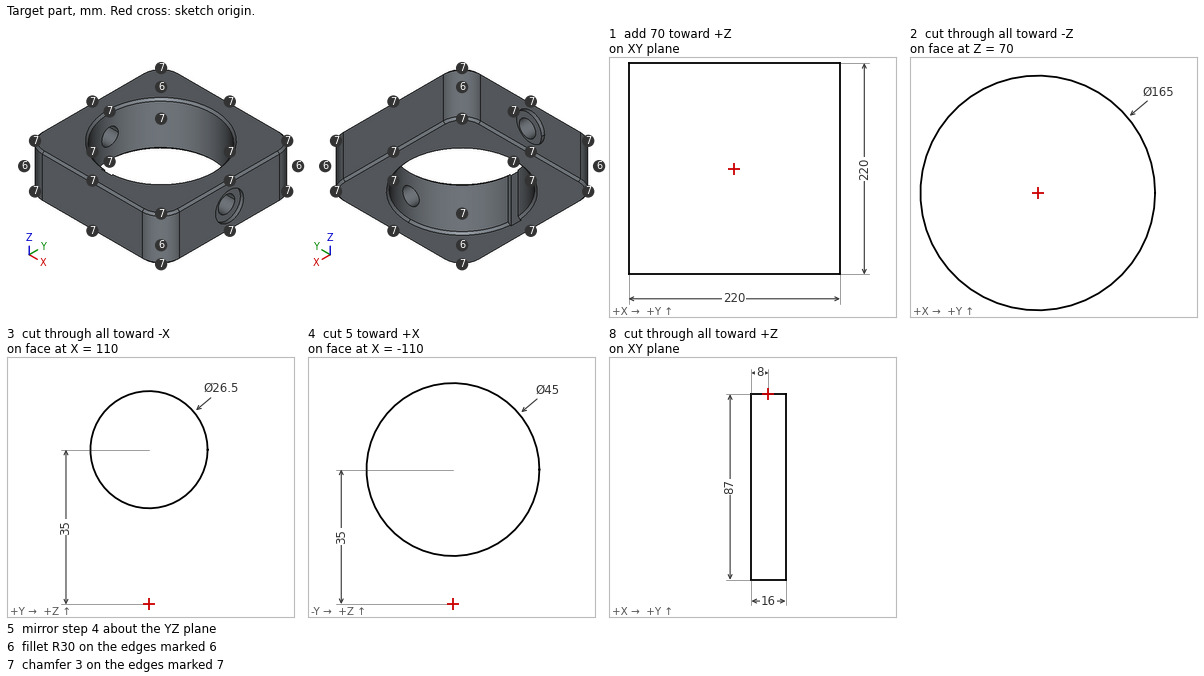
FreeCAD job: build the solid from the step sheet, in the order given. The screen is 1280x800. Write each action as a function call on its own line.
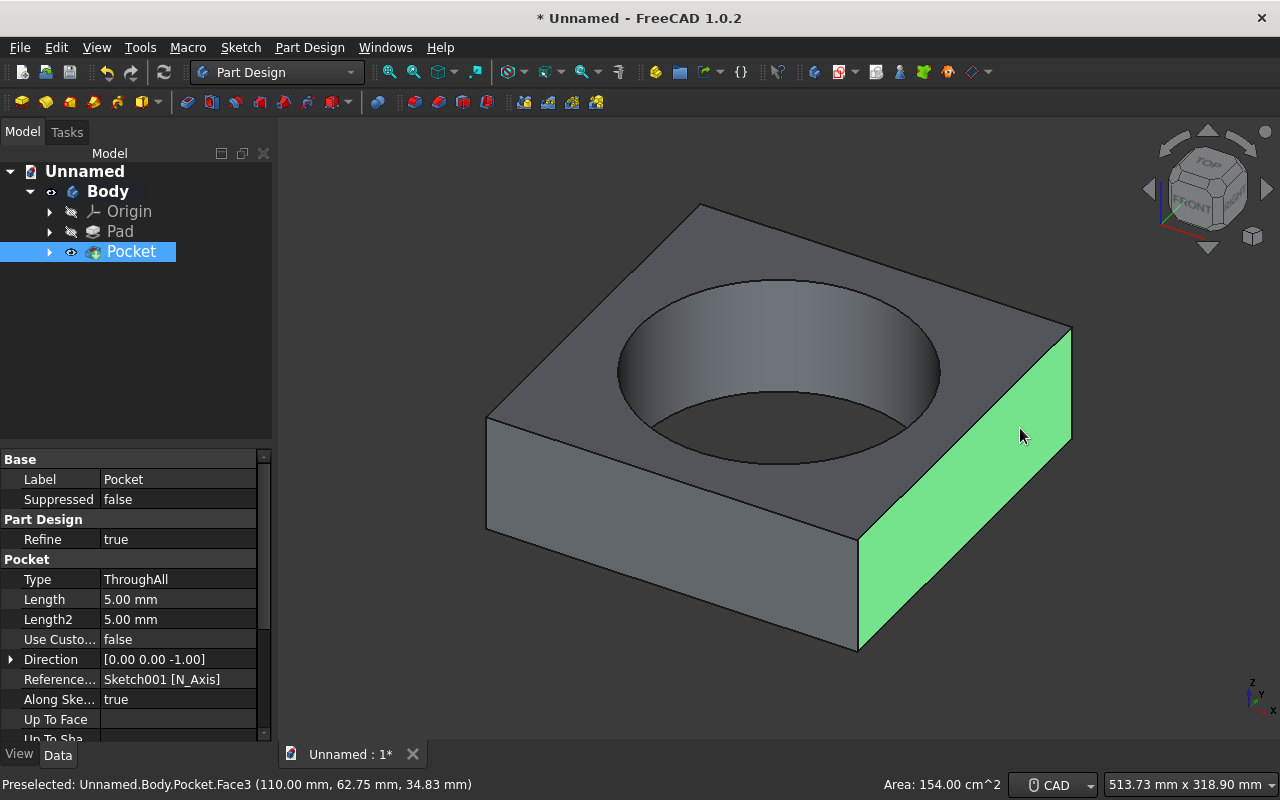
click(840, 72)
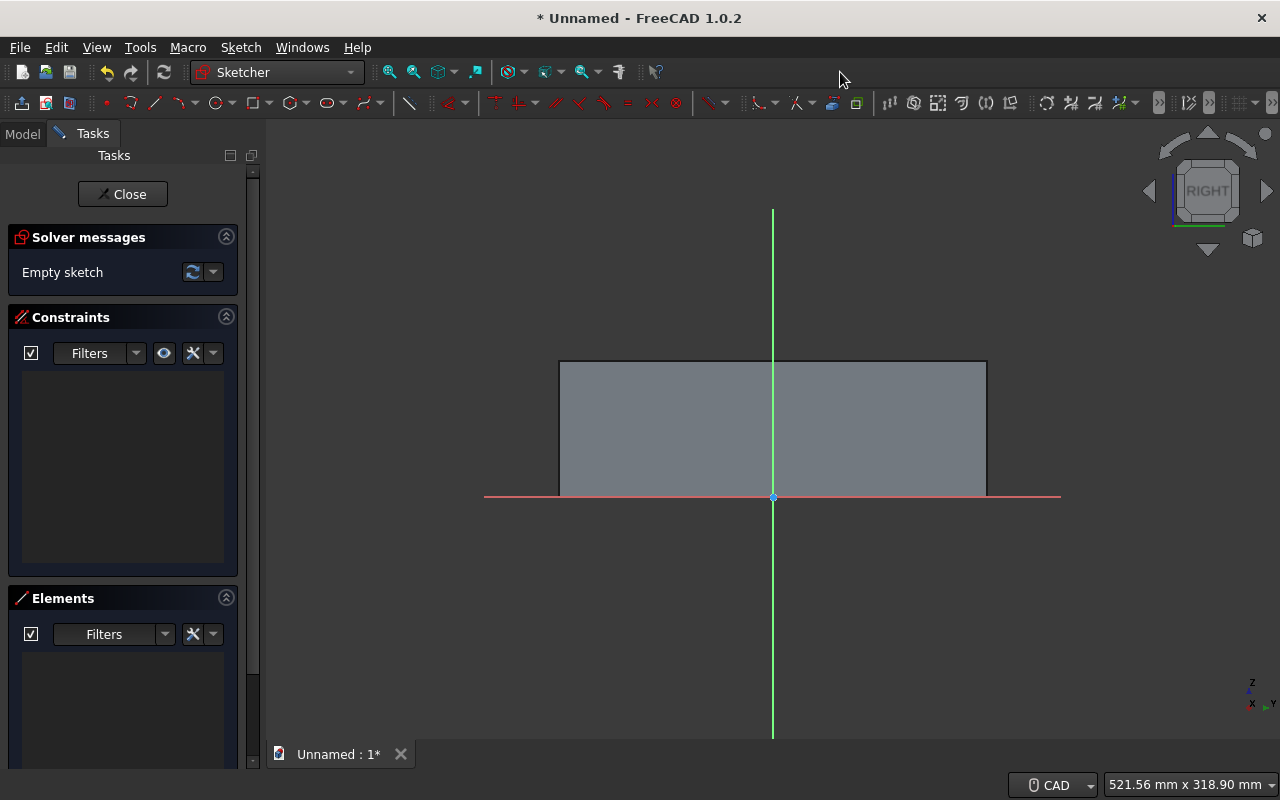
scroll(795, 457, up, 7)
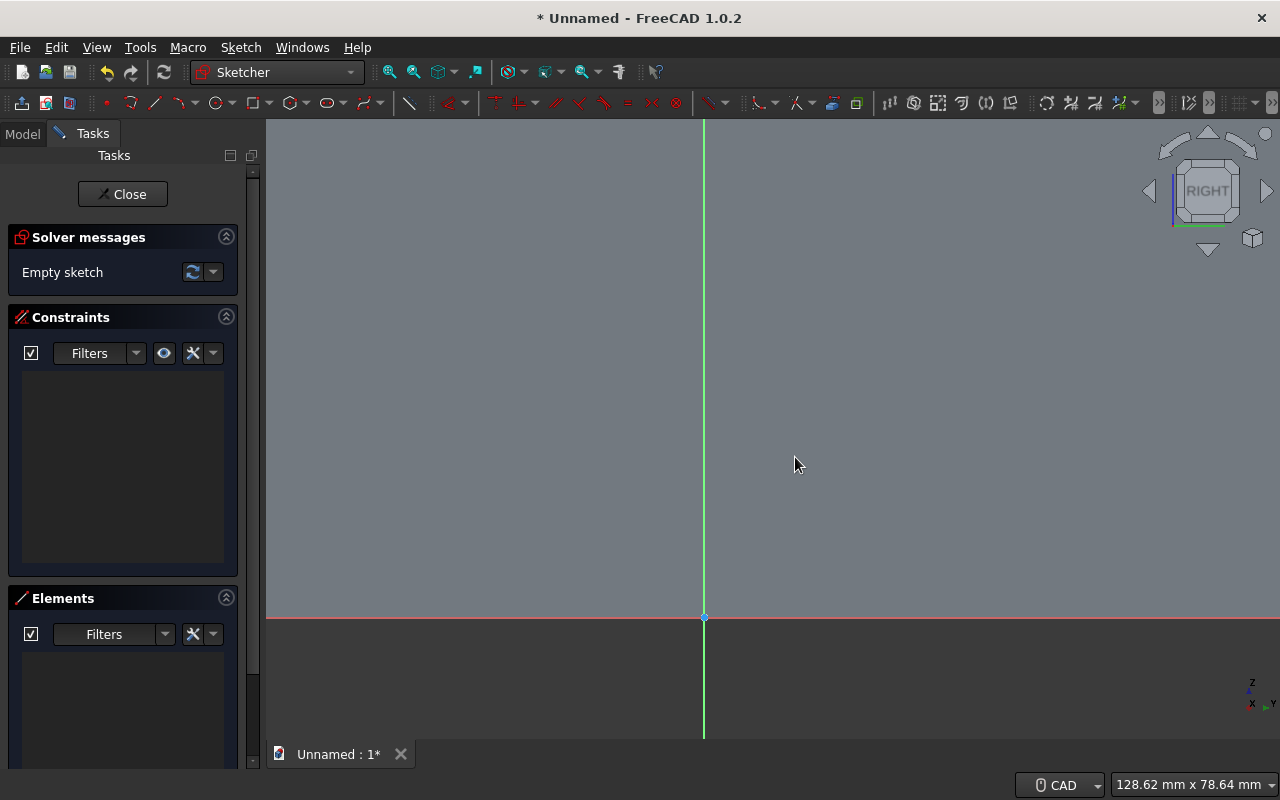
click(216, 104)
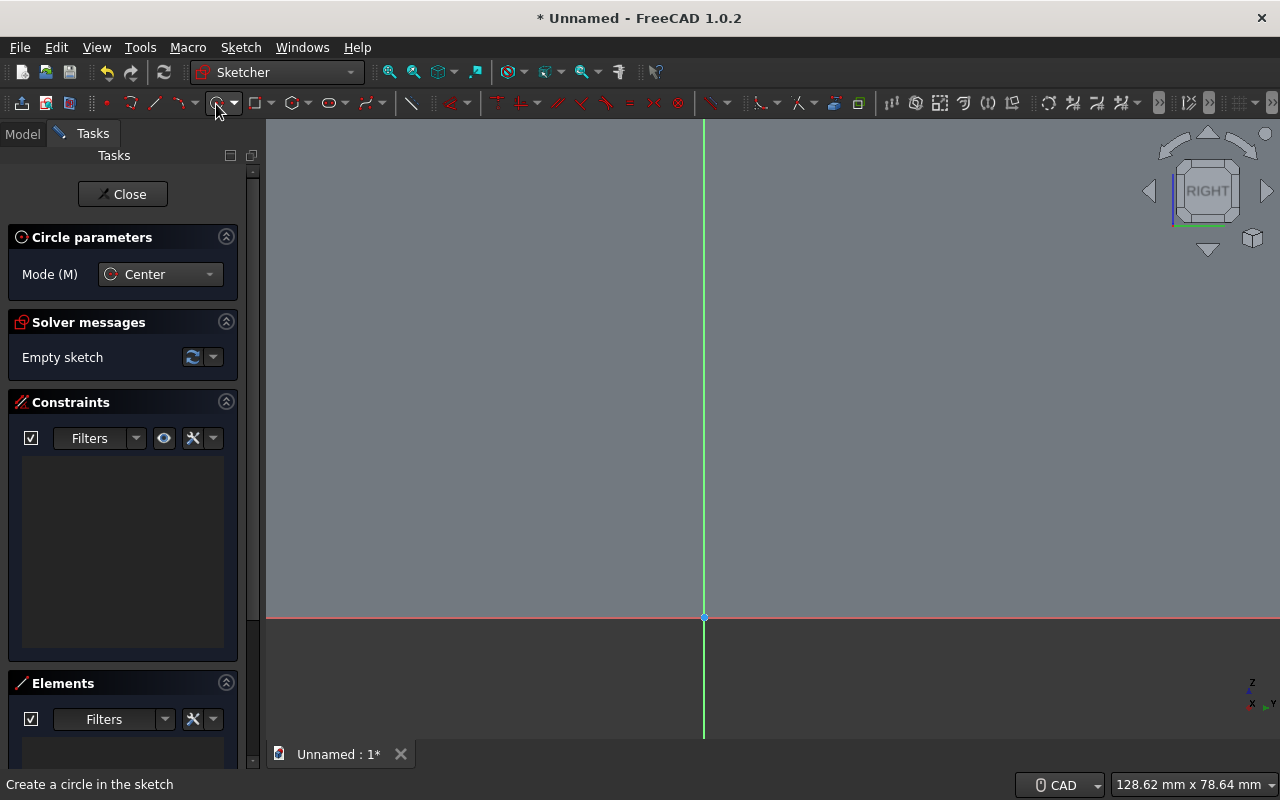
click(704, 342)
click(778, 268)
key(Escape)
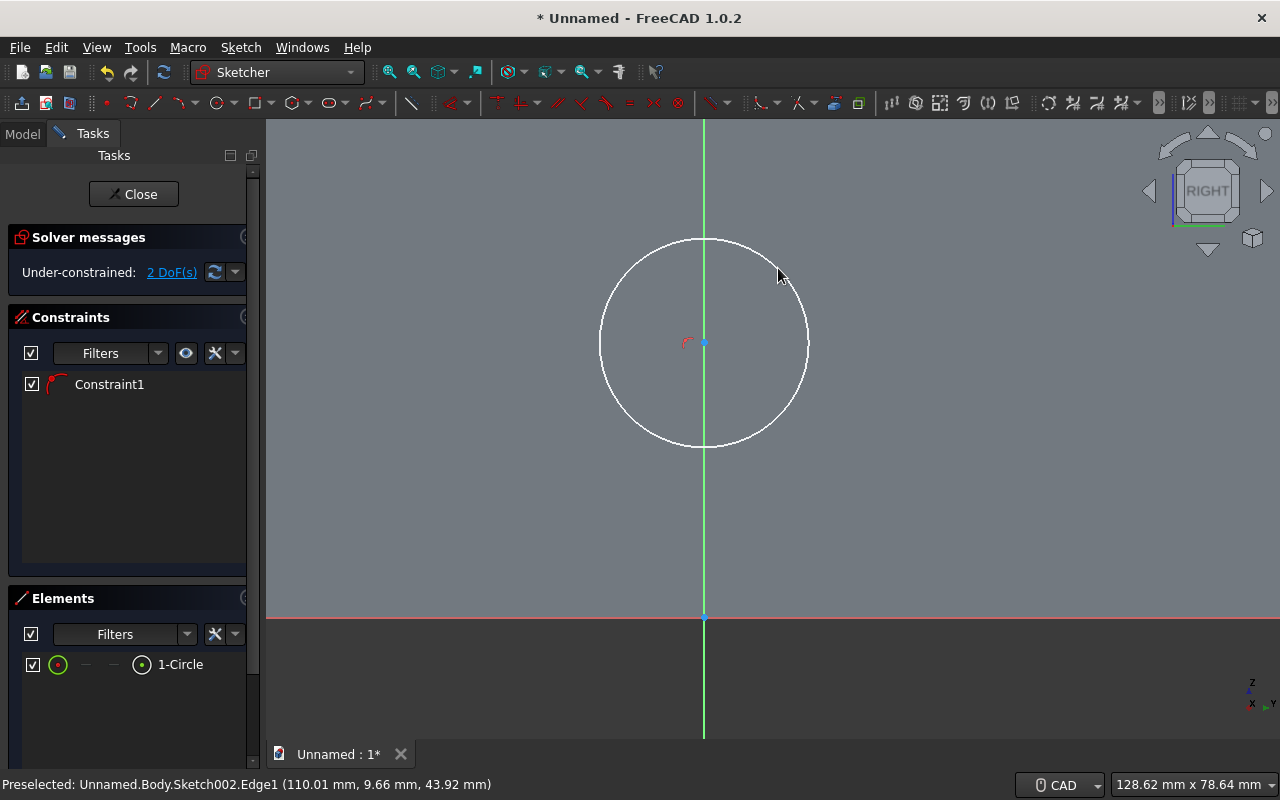
key(d)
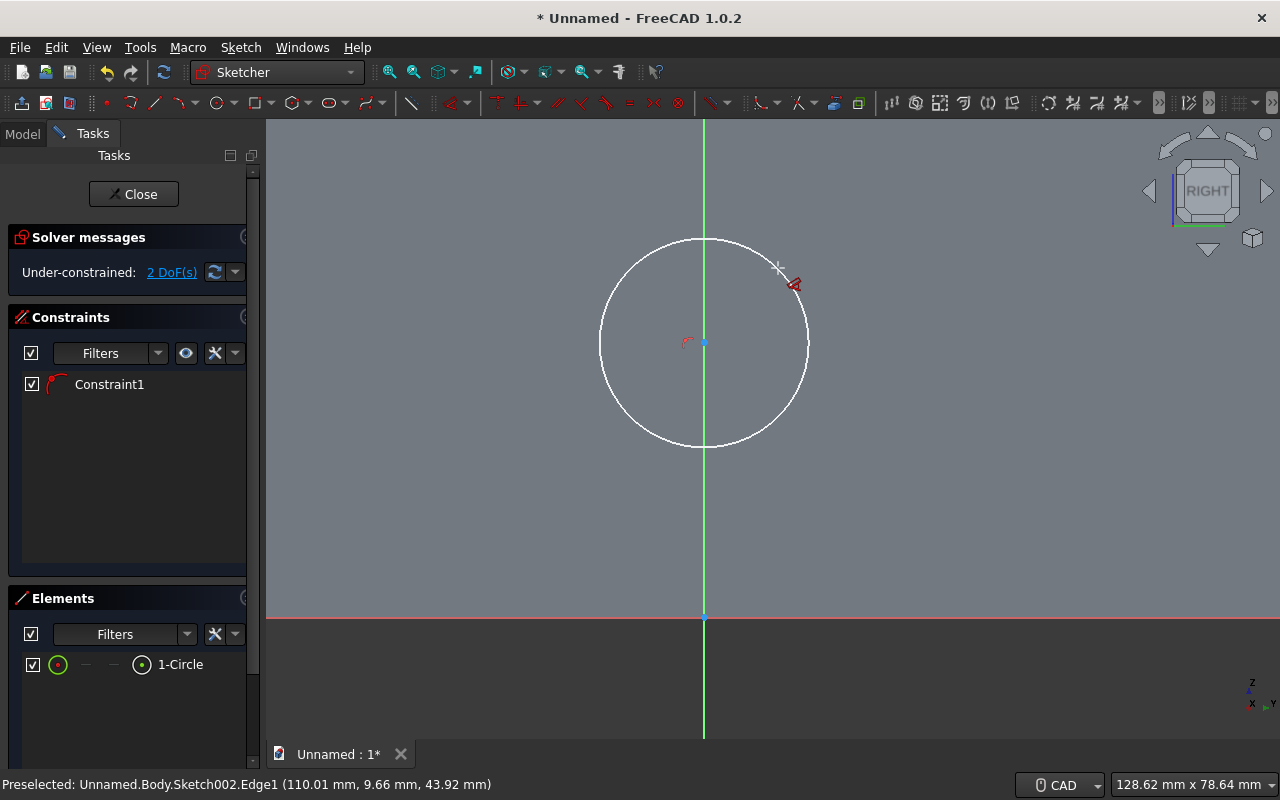
click(778, 269)
click(801, 246)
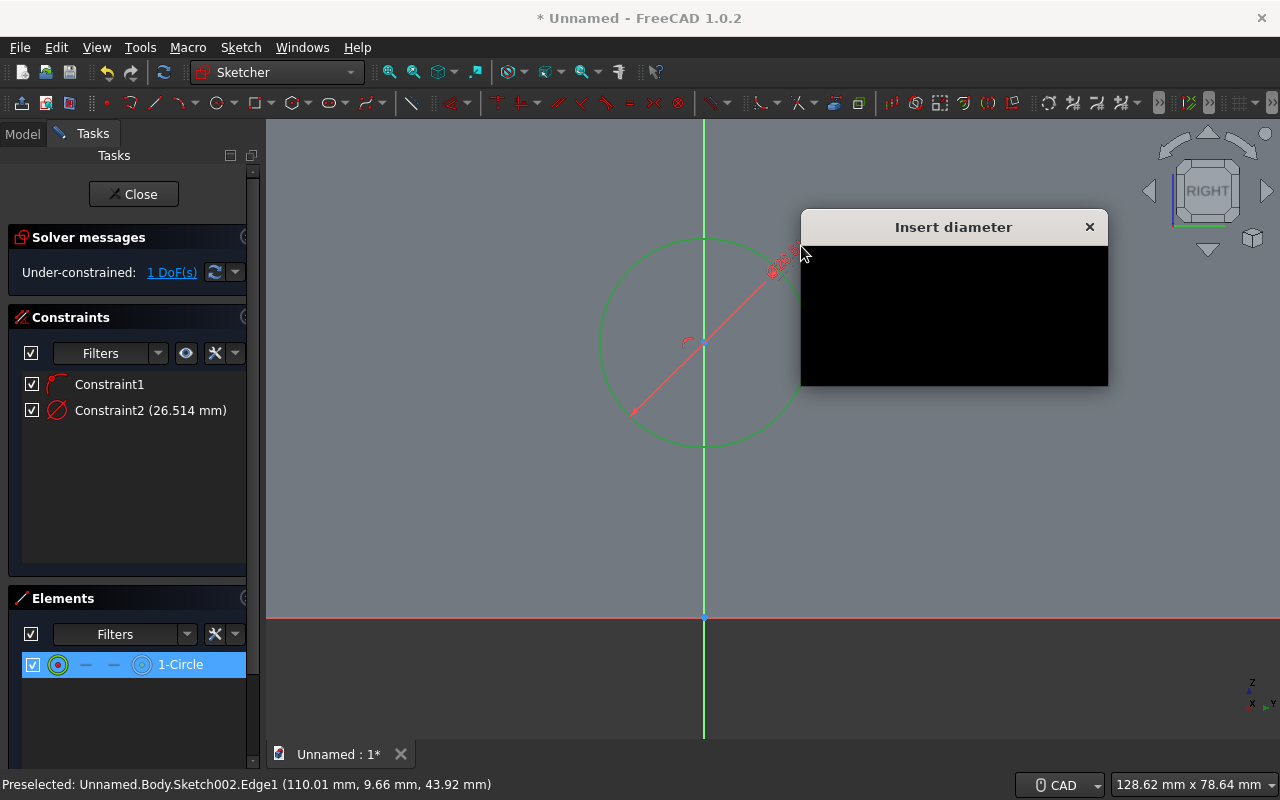
text(26.5)
key(Return)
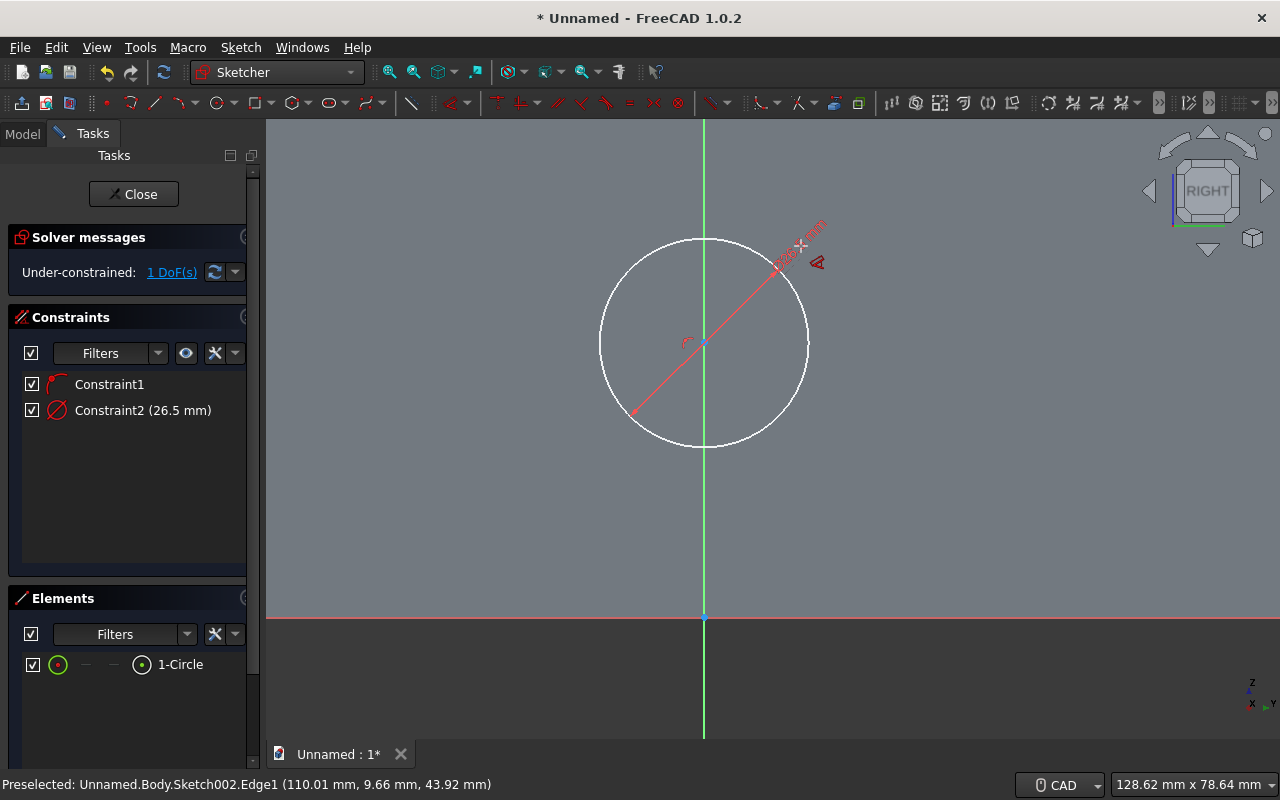
click(704, 343)
click(738, 480)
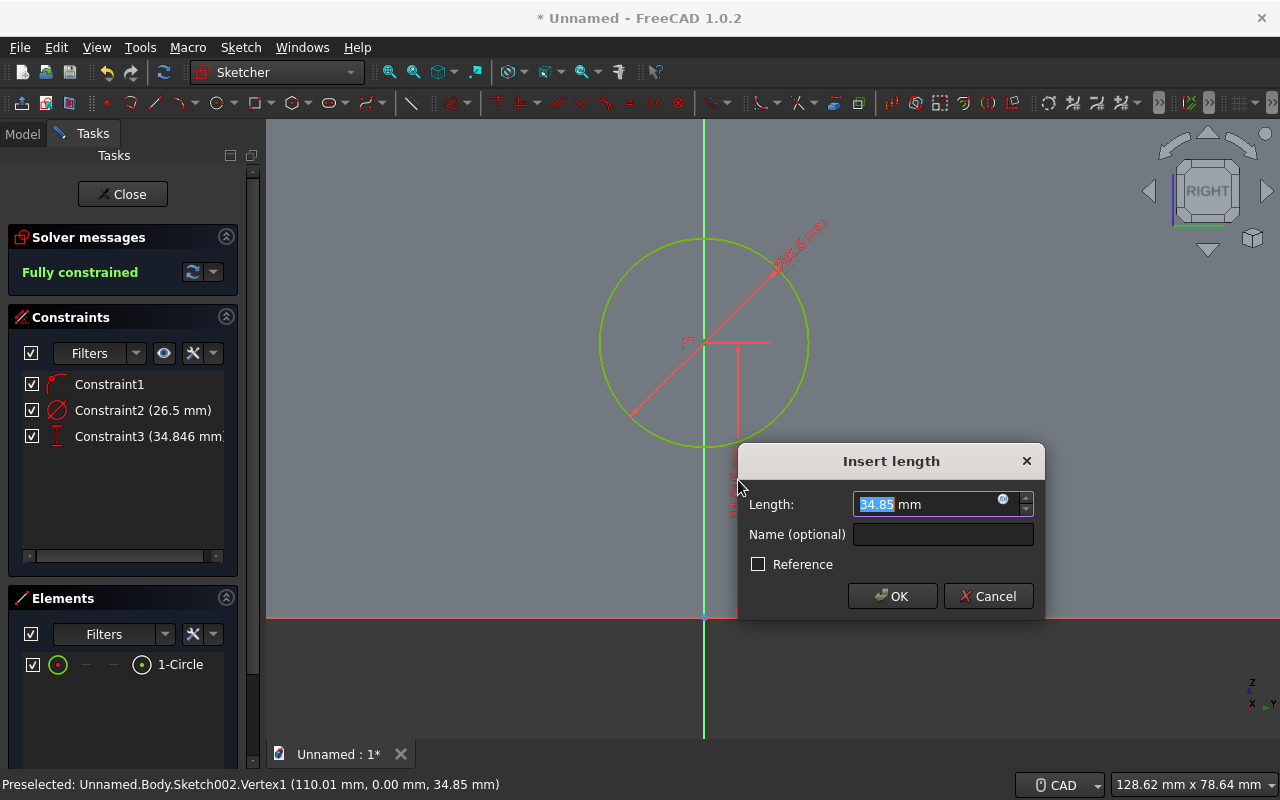
text(35)
key(Return)
key(Escape)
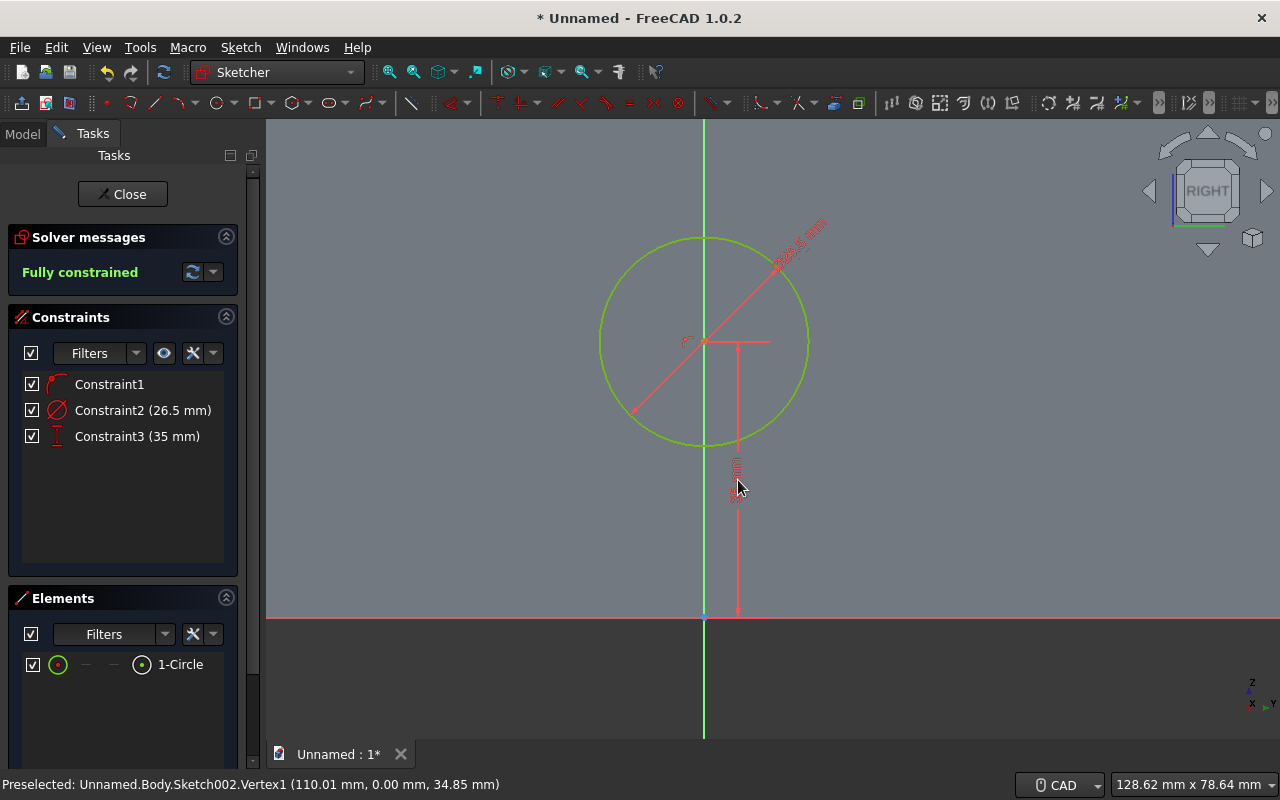
click(123, 194)